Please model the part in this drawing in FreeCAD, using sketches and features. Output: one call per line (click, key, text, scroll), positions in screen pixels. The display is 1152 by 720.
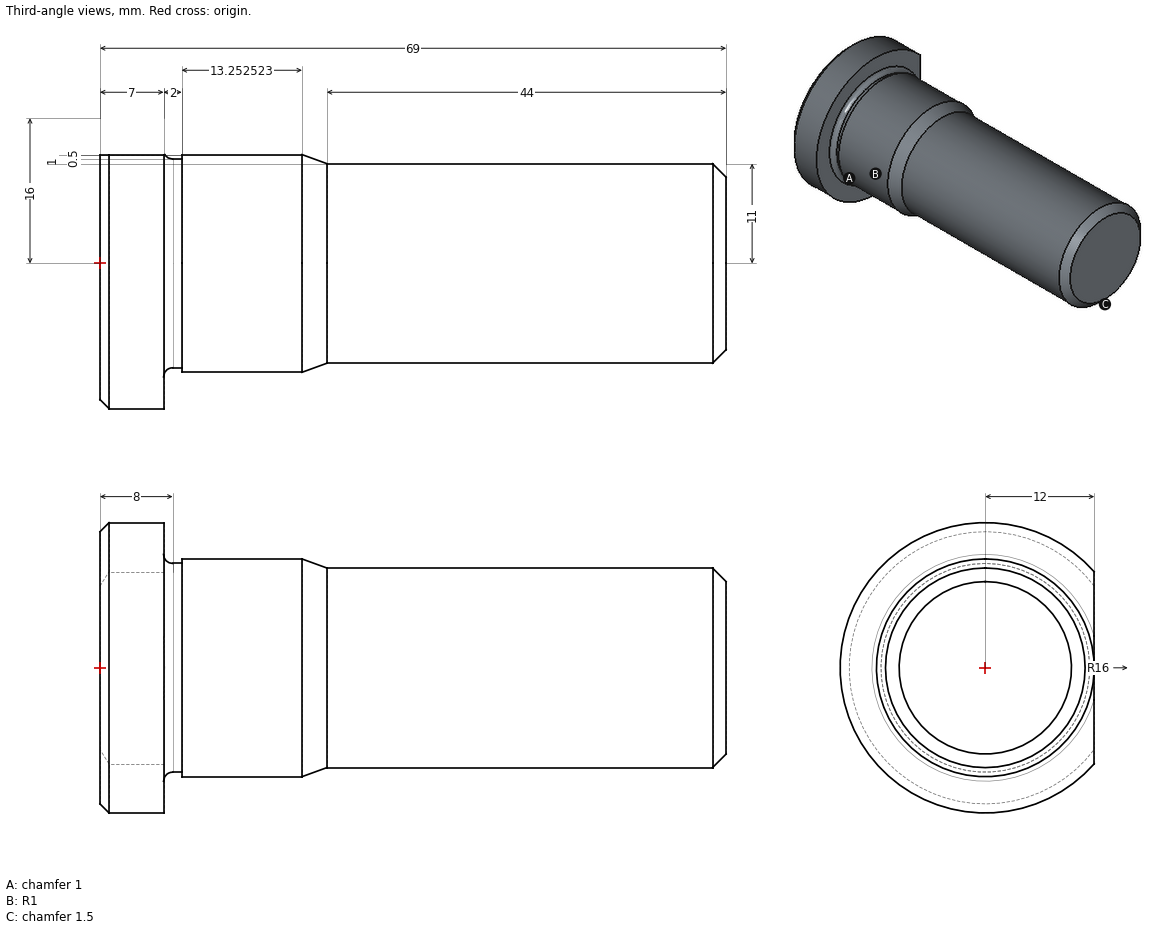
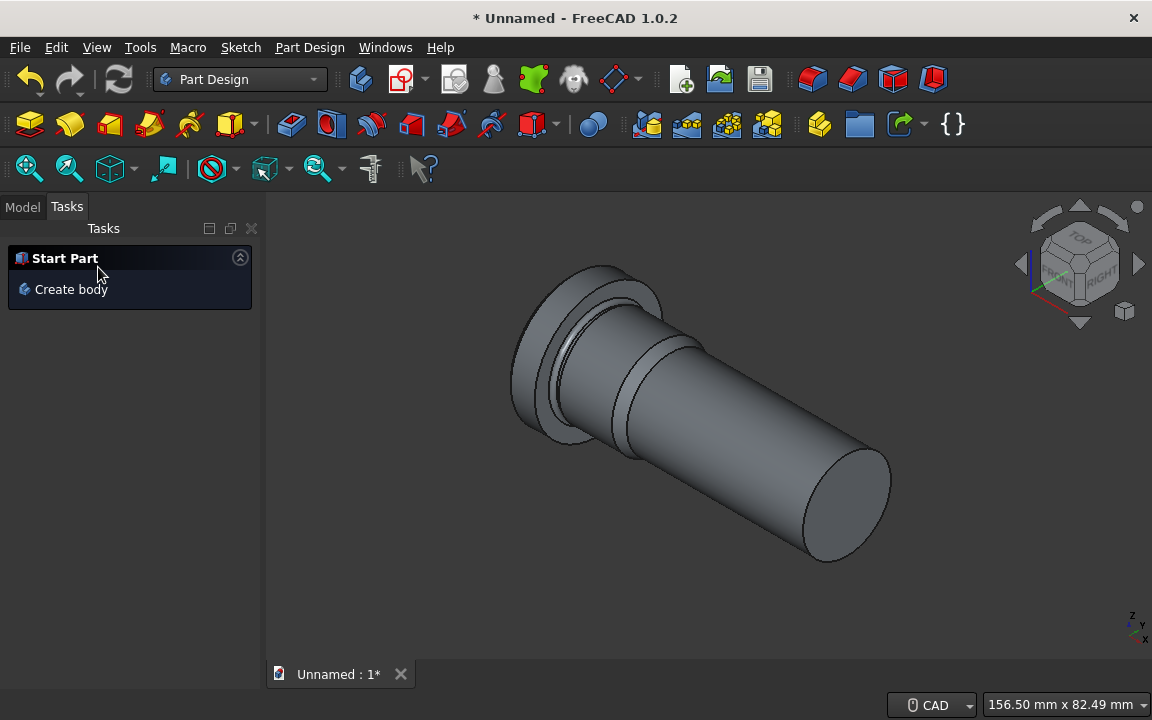
click(803, 530)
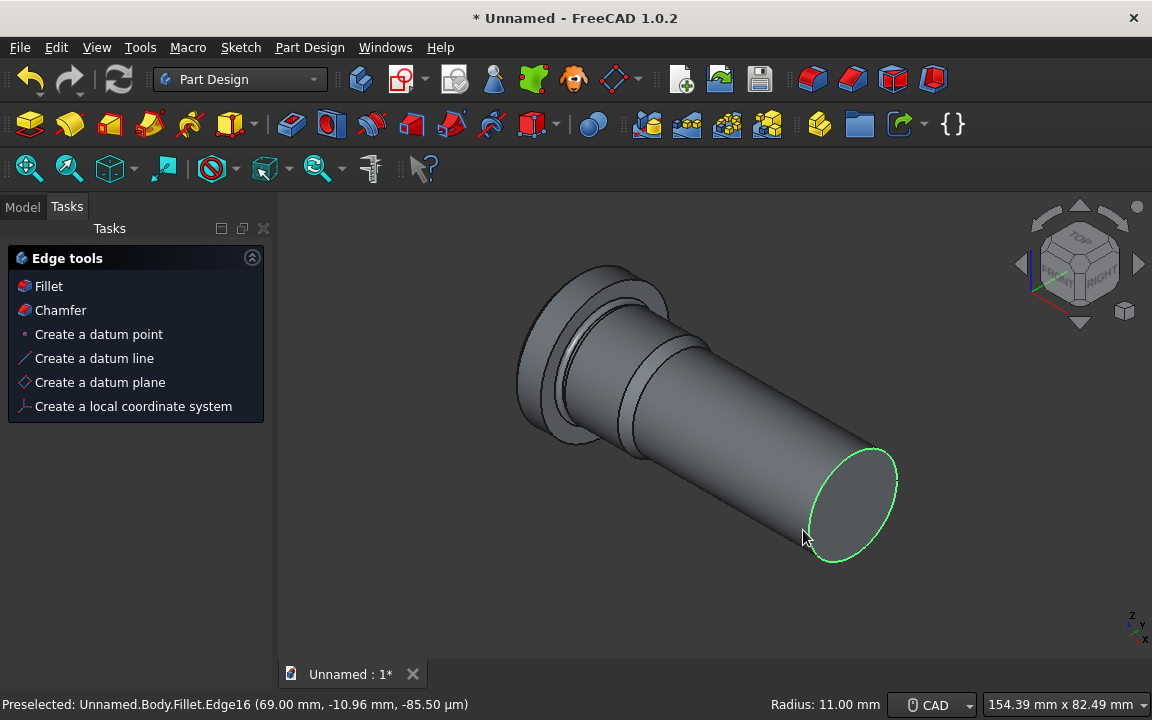
click(854, 80)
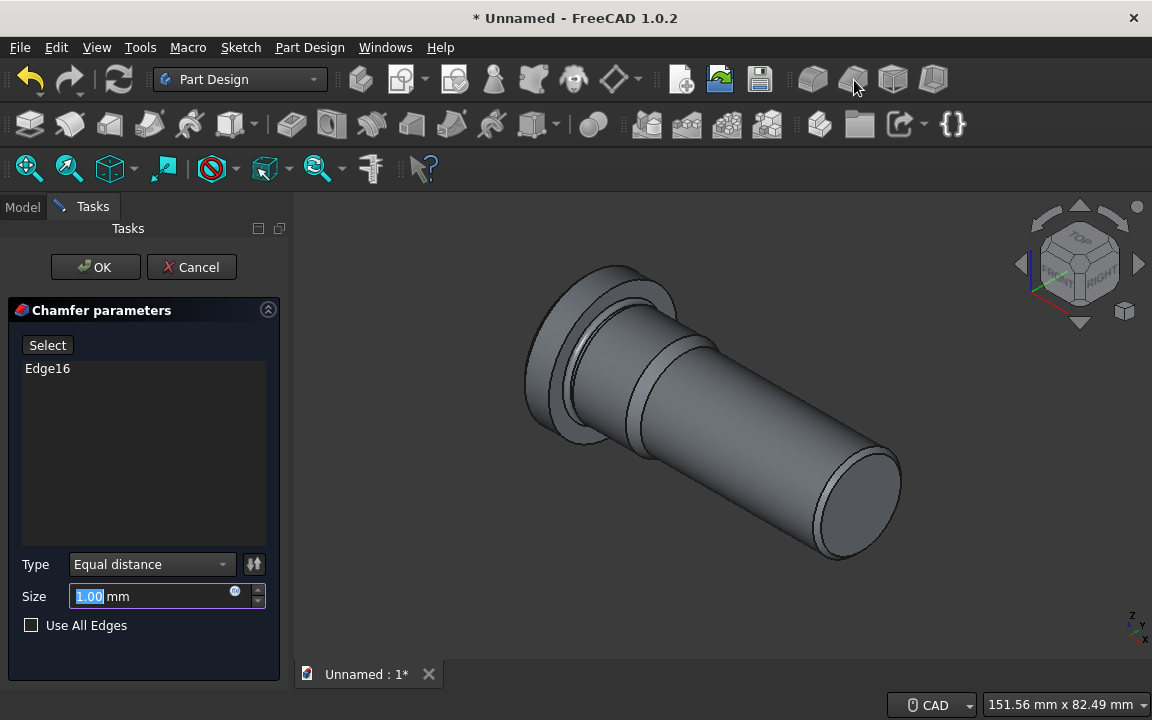
text(1.5)
key(Tab)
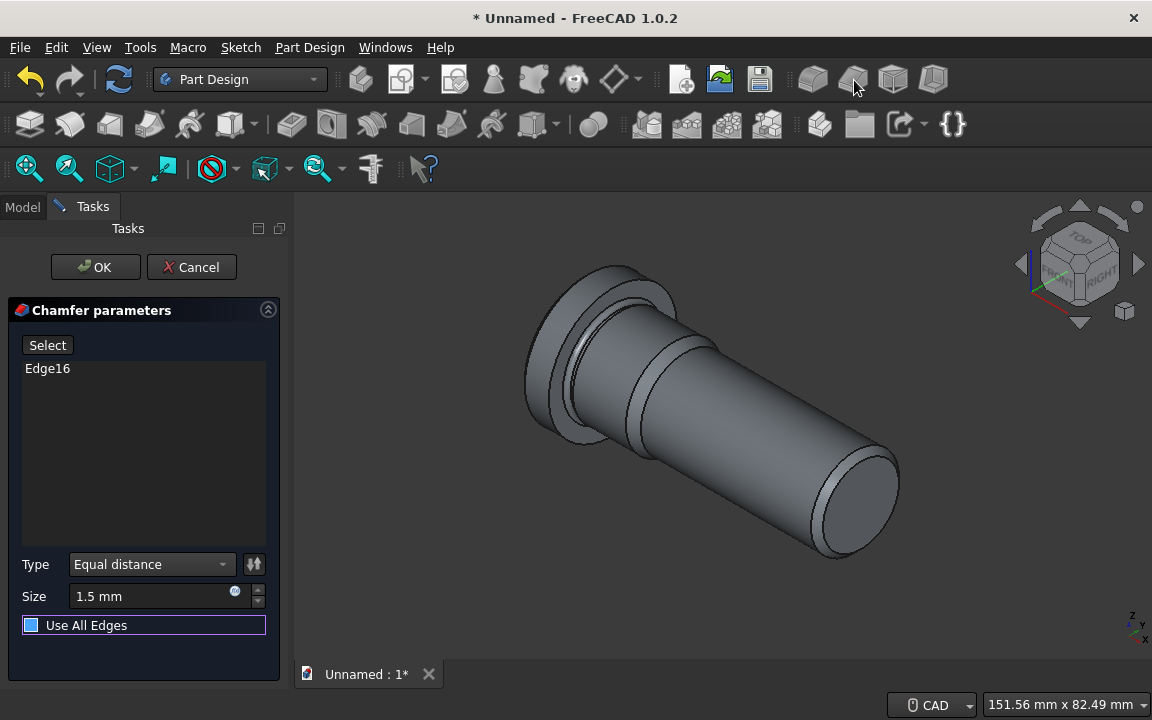
click(96, 267)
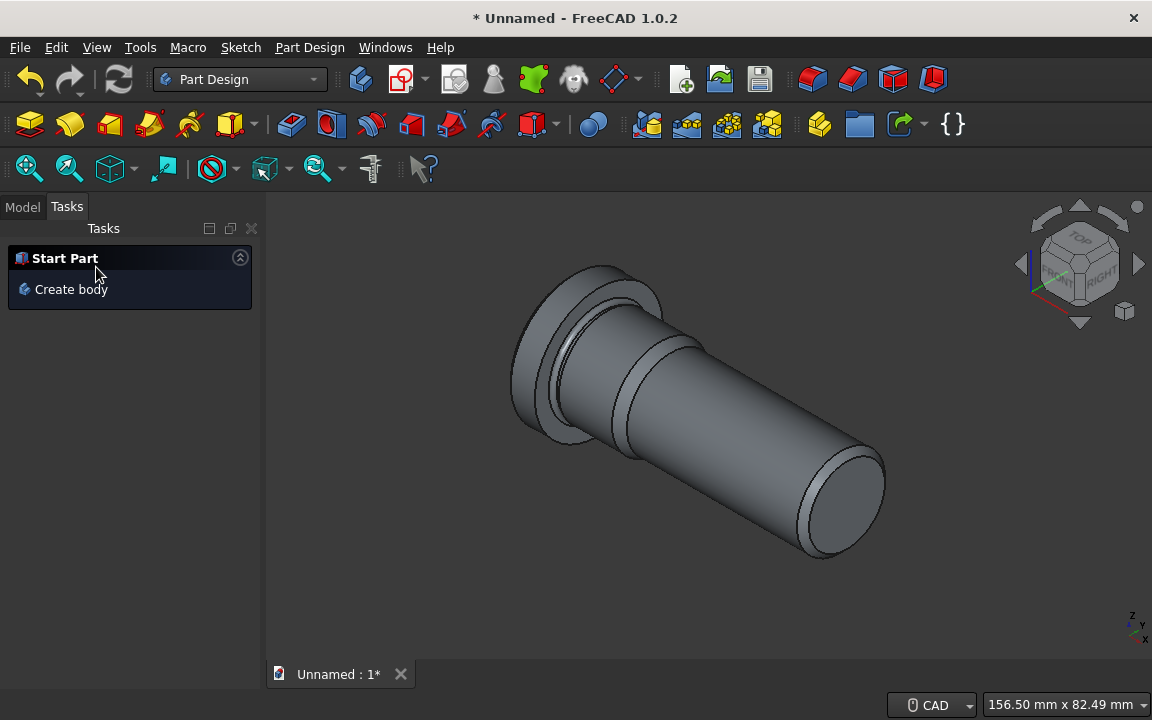
click(23, 206)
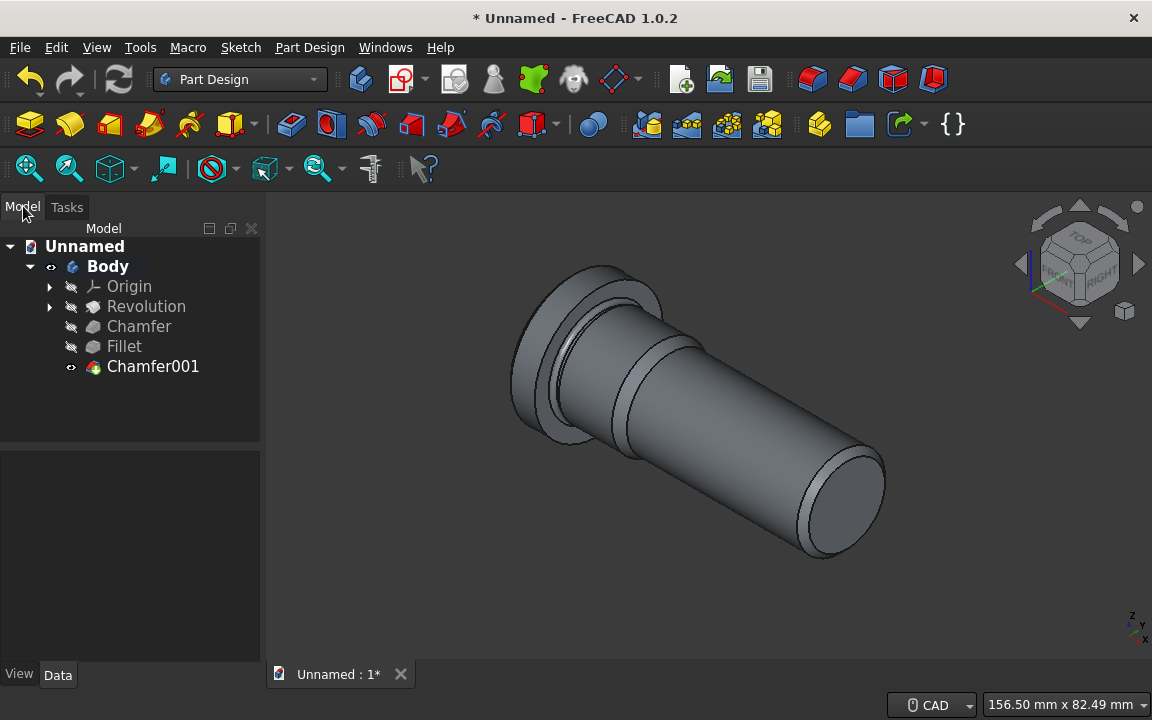
click(50, 287)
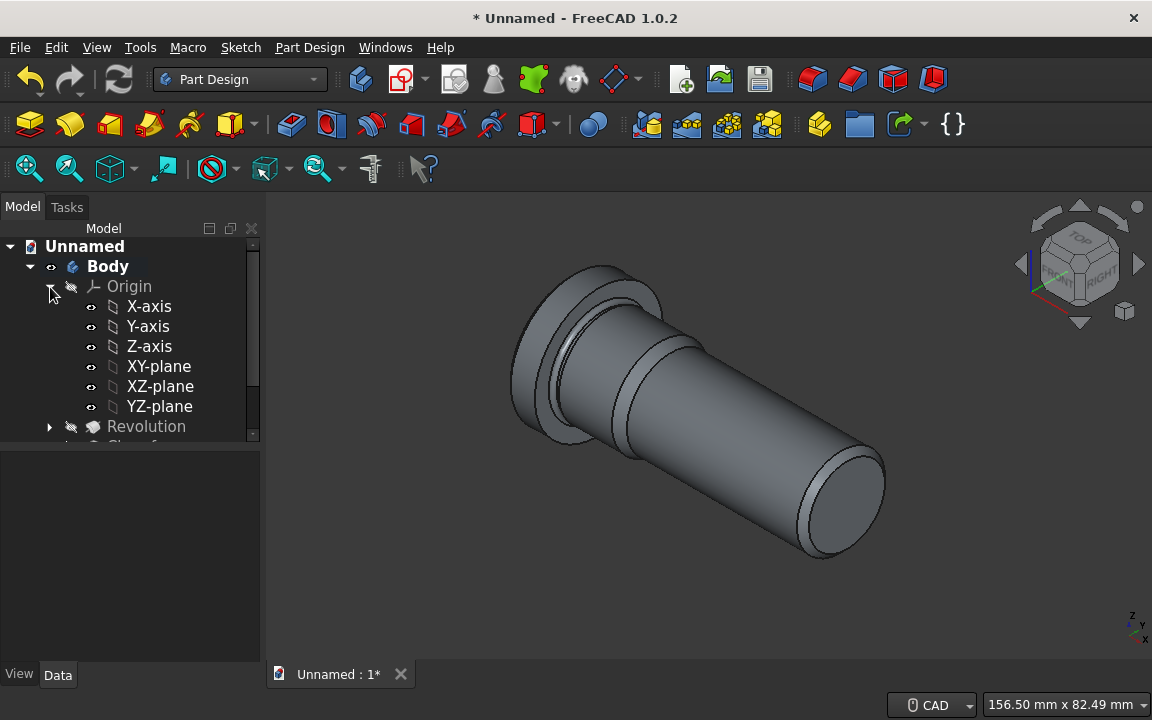
click(136, 407)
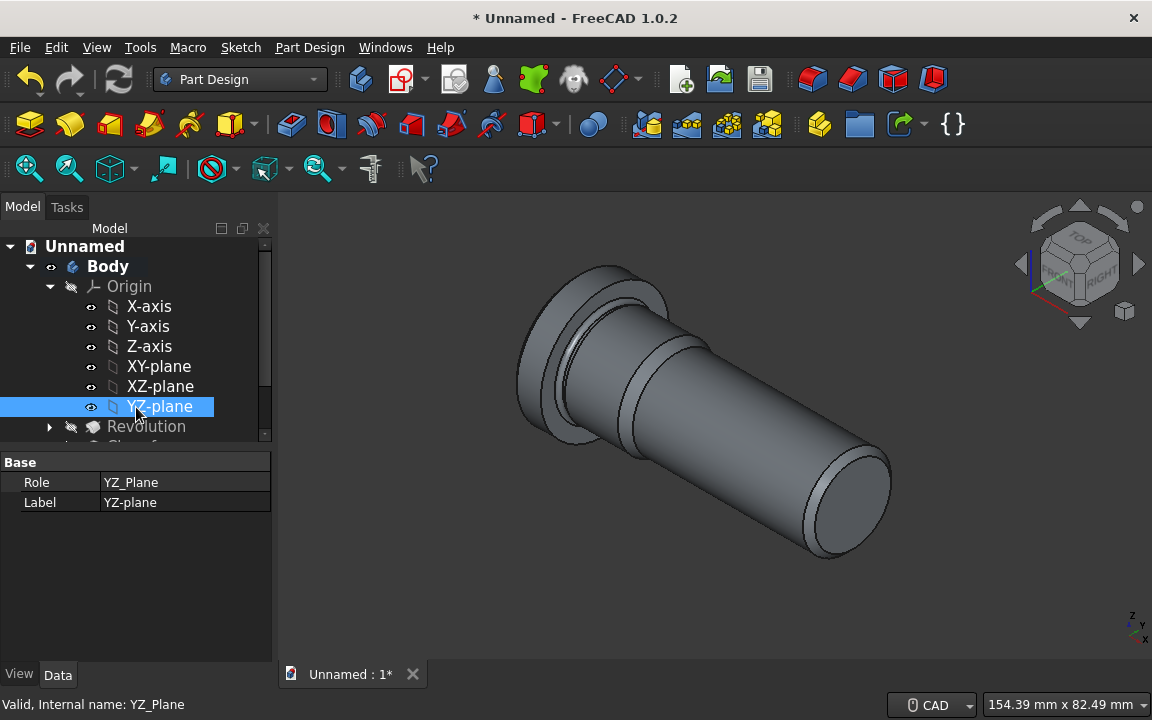
click(614, 80)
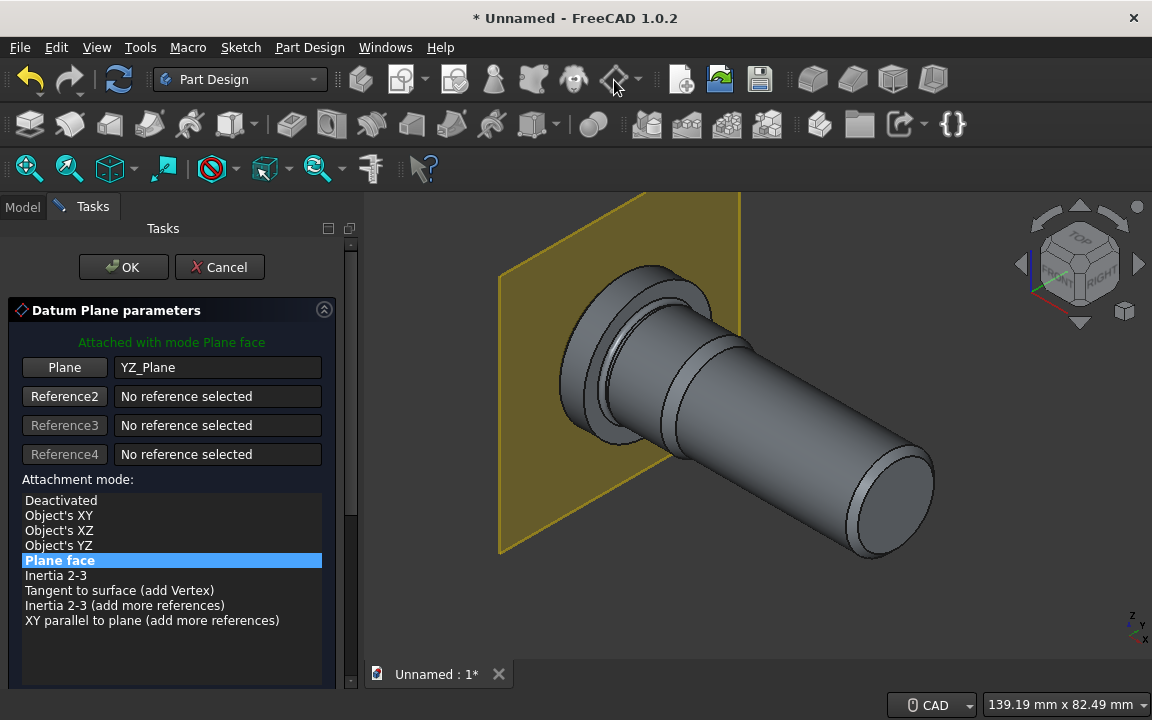
scroll(351, 463, down, 3)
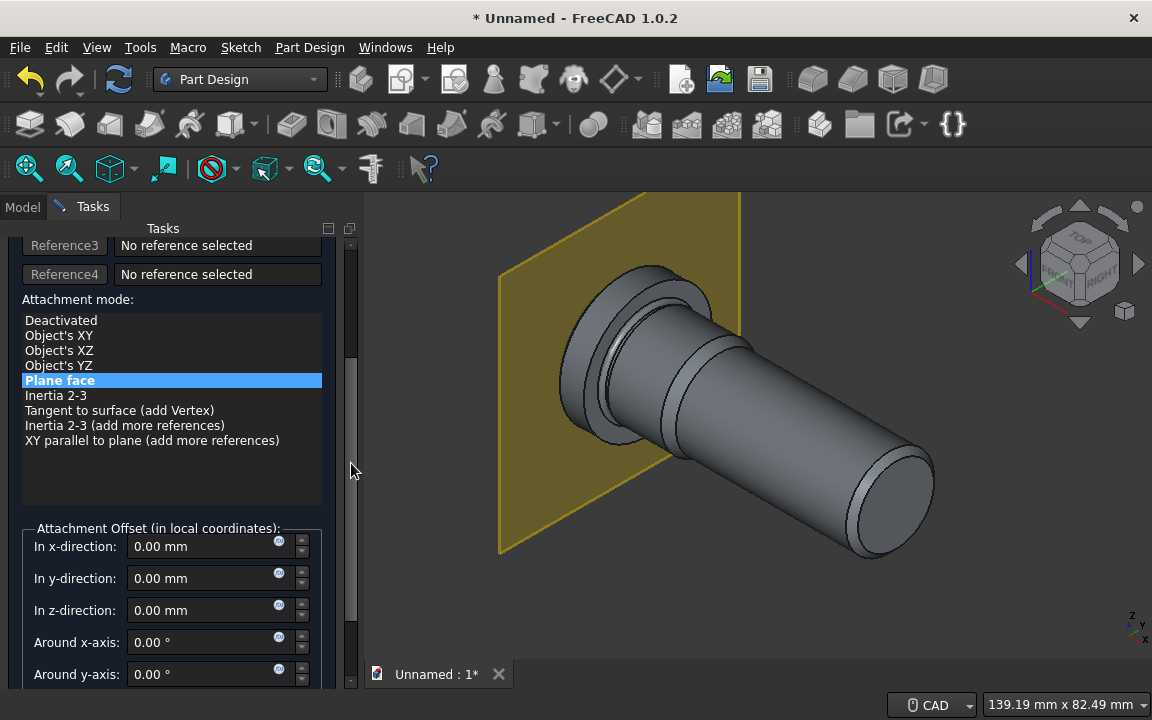
triple_click(210, 610)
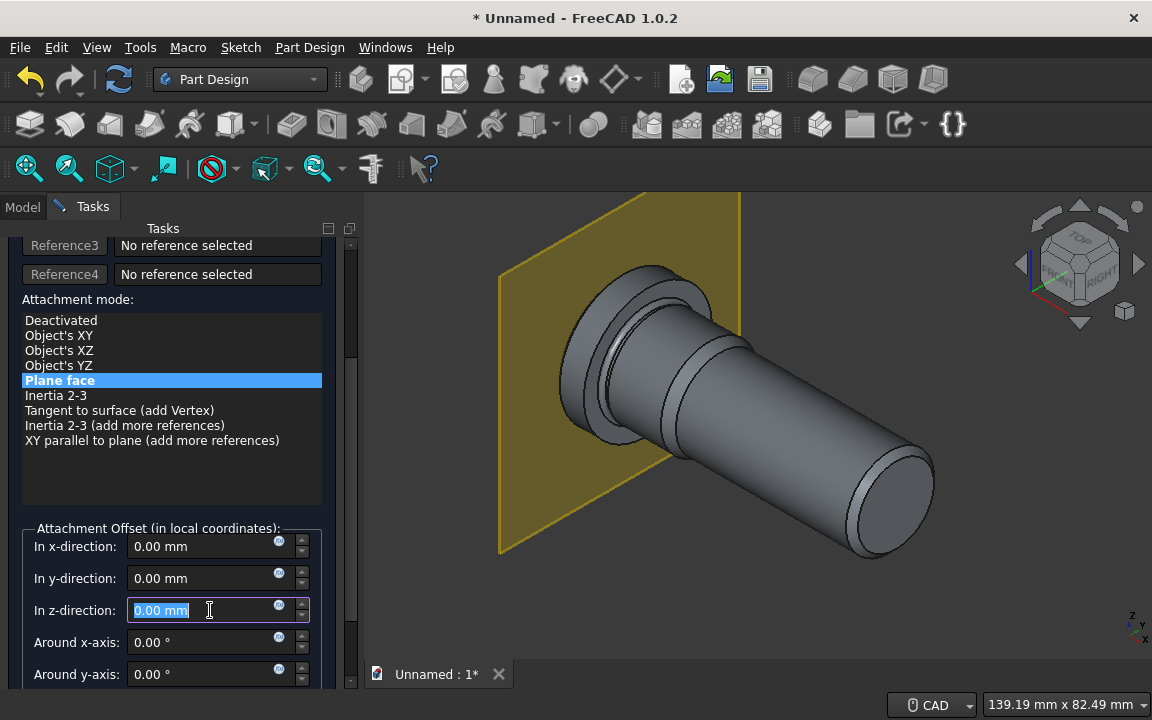
text(8)
key(Tab)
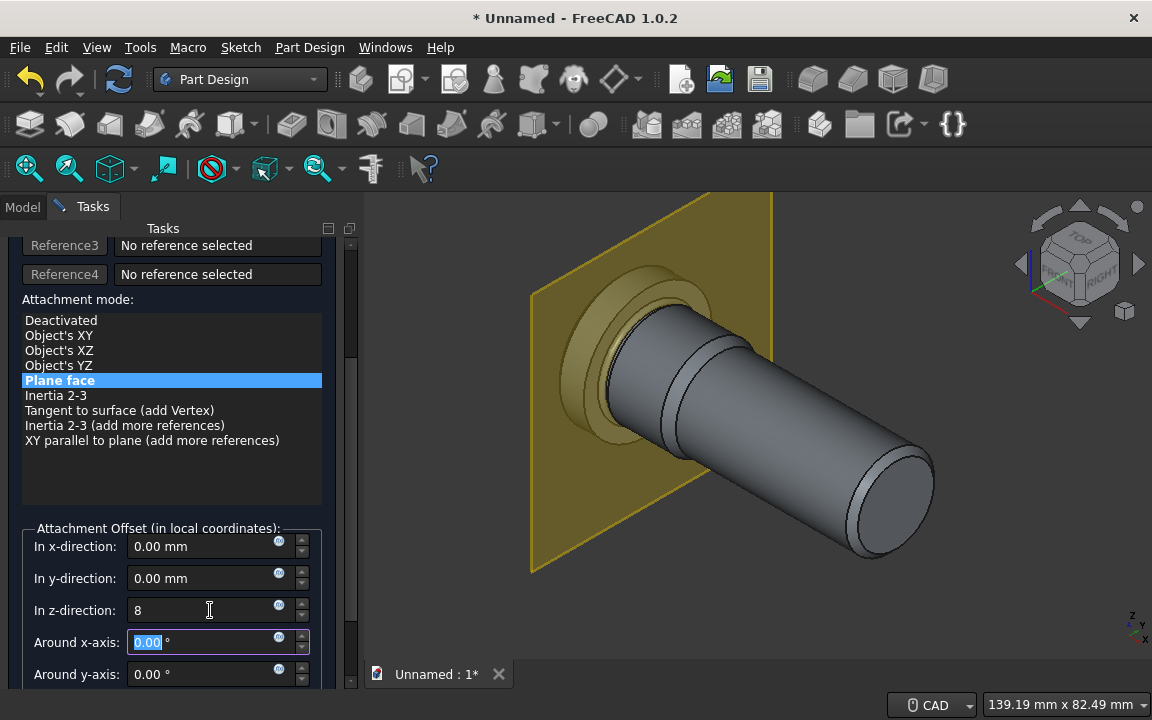
scroll(351, 463, up, 4)